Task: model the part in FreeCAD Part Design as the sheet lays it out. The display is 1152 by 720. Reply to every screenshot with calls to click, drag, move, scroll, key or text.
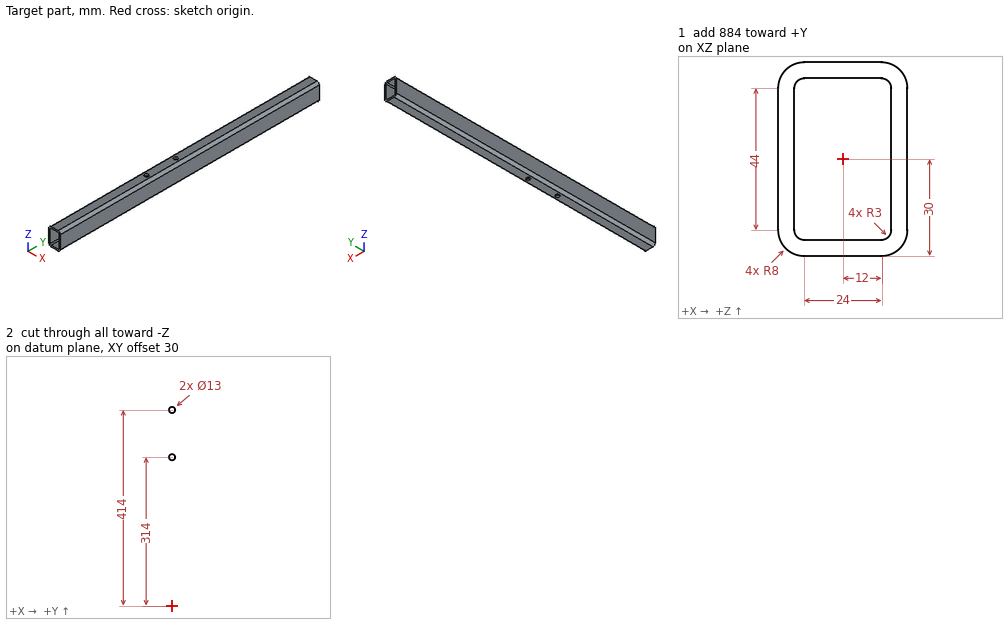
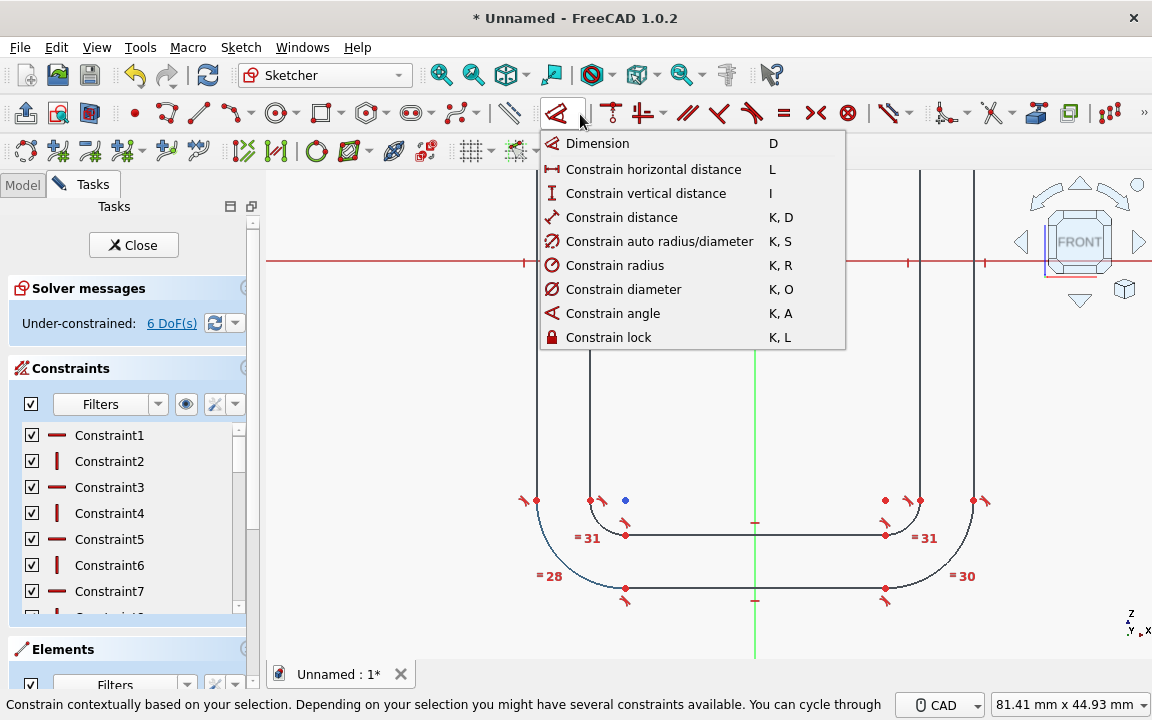
click(693, 265)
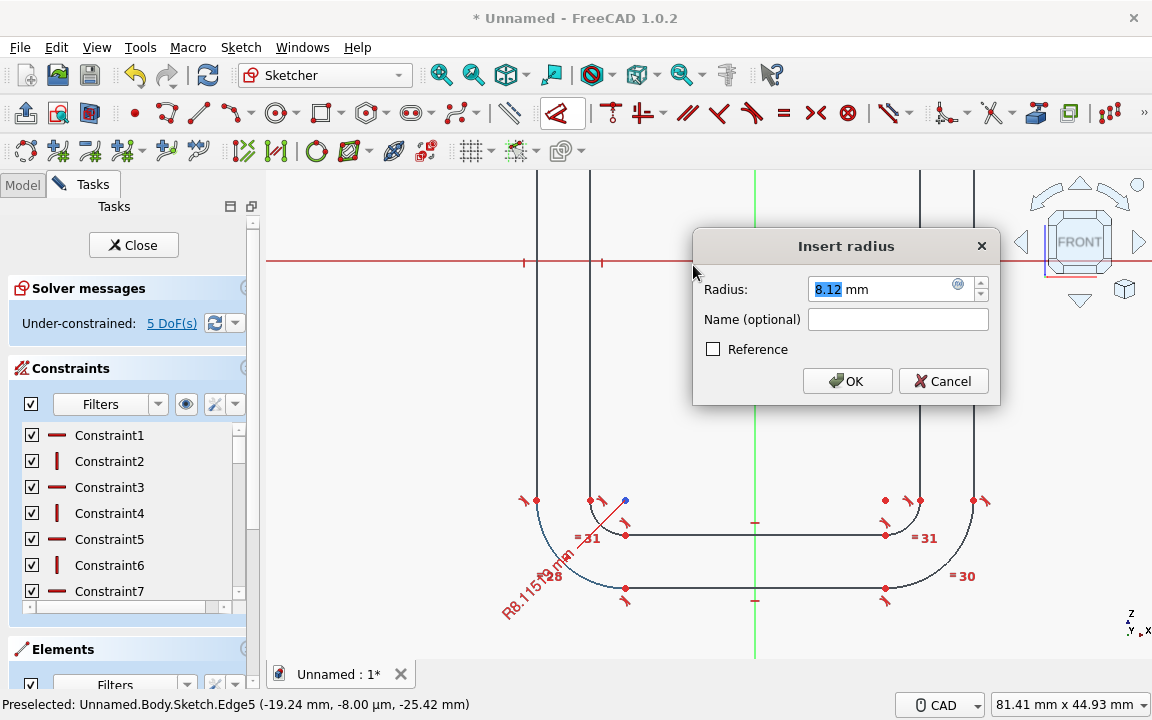
text(8)
key(Return)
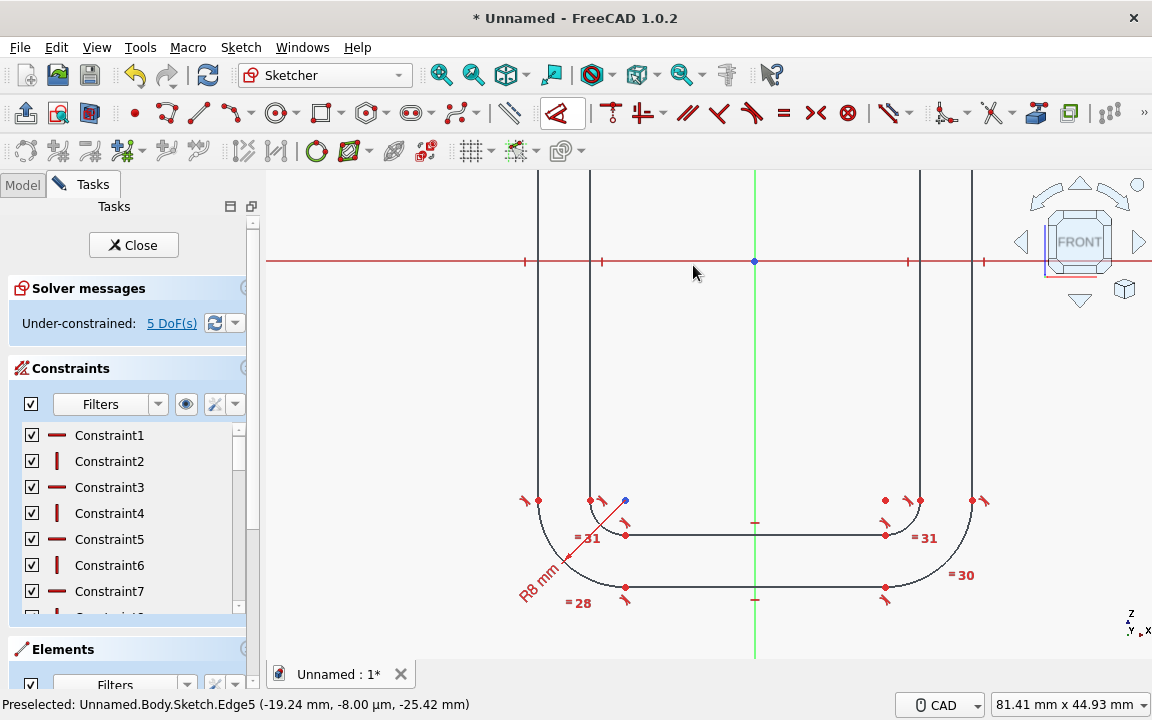
click(901, 531)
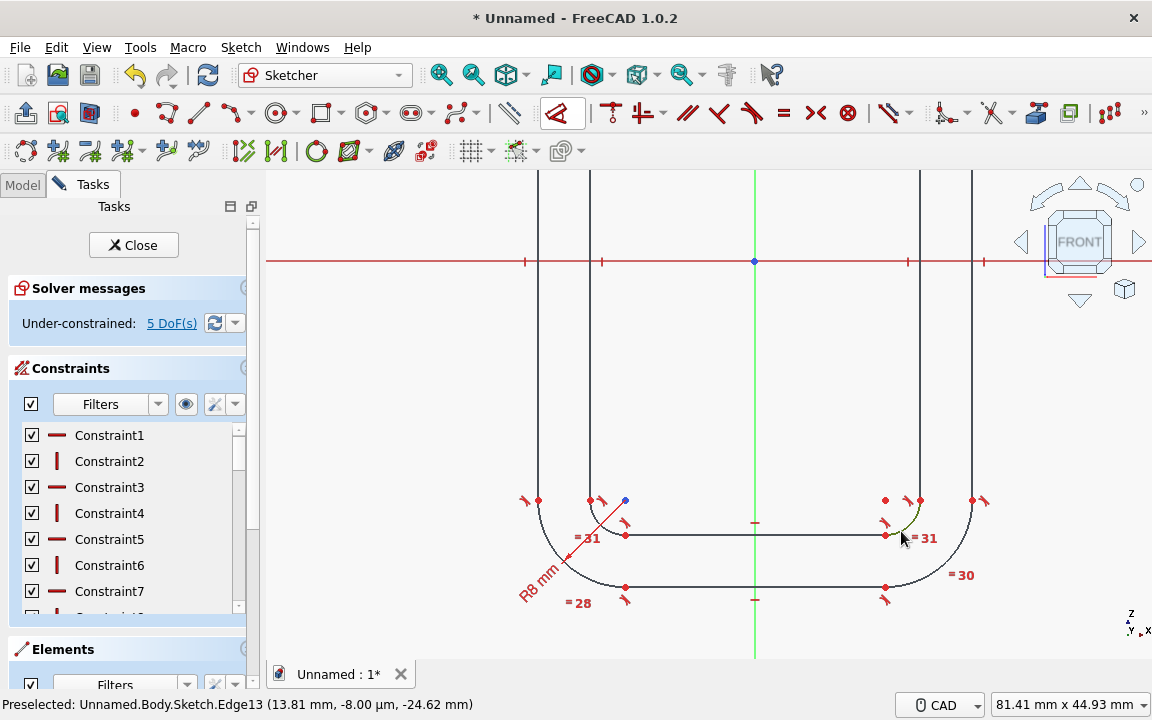
key(k)
key(r)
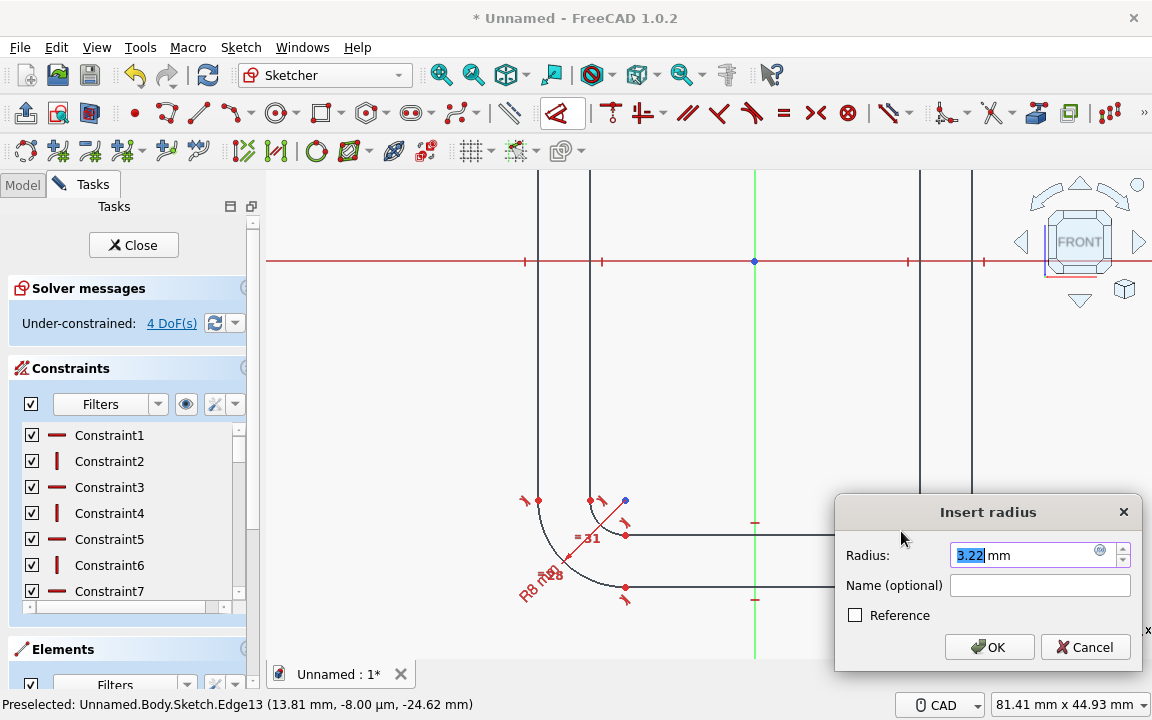
text(3)
key(Return)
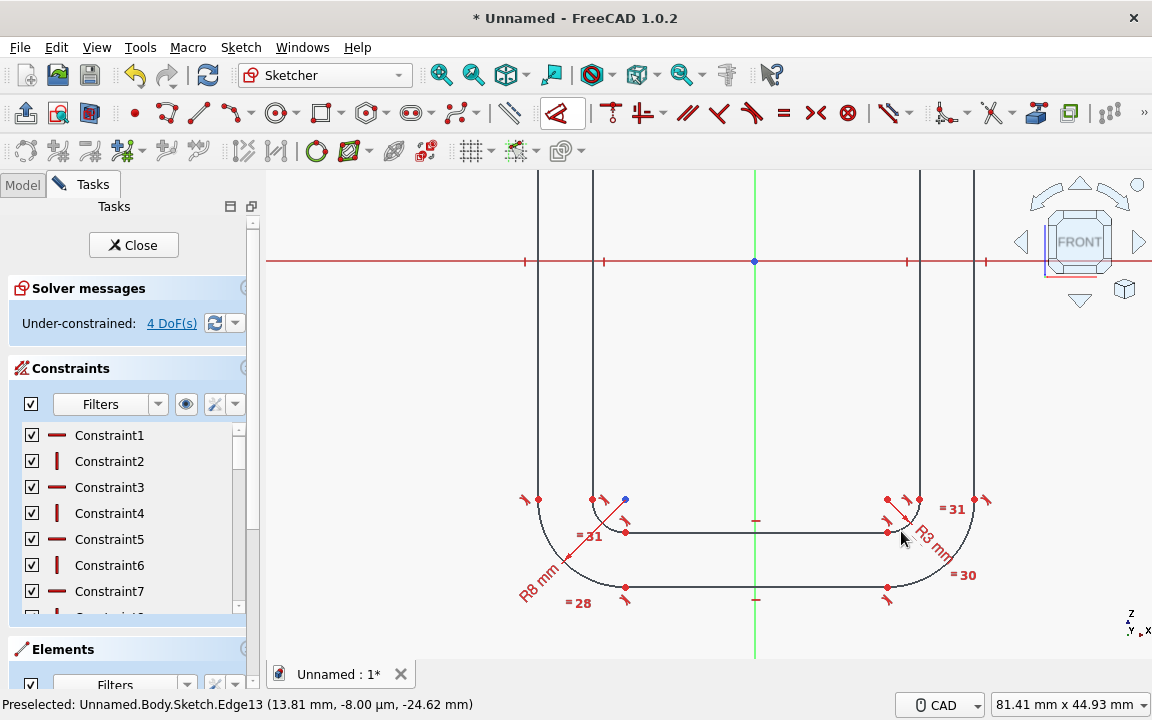
click(809, 587)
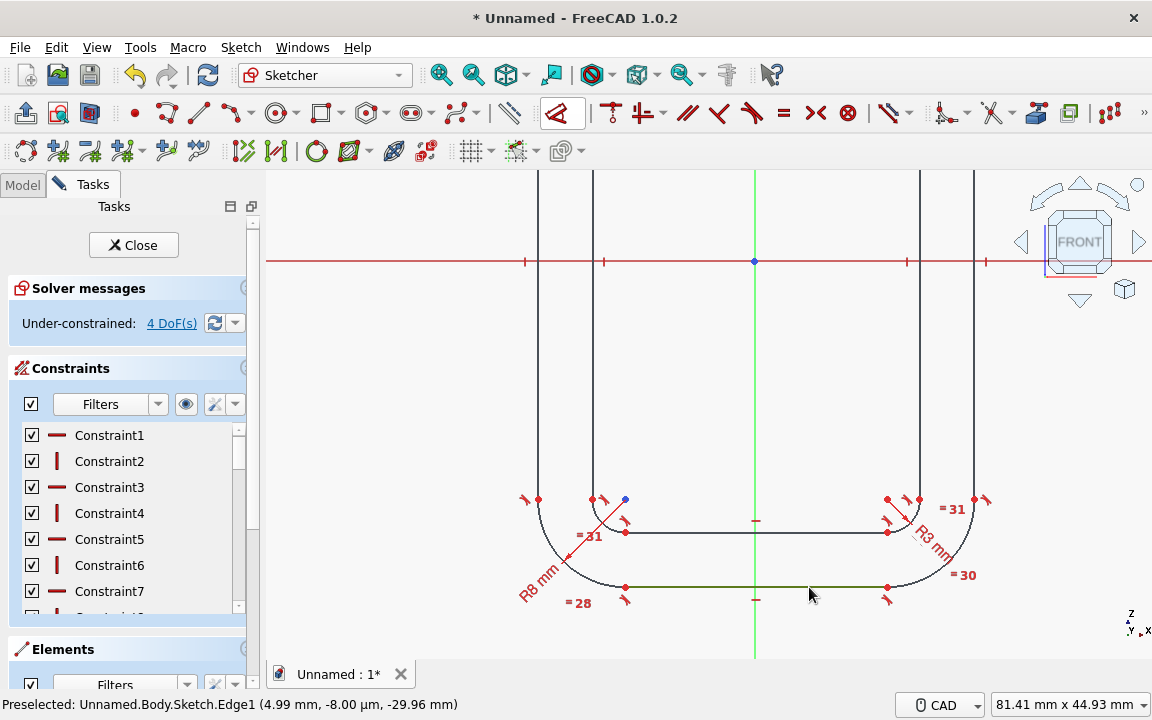
key(l)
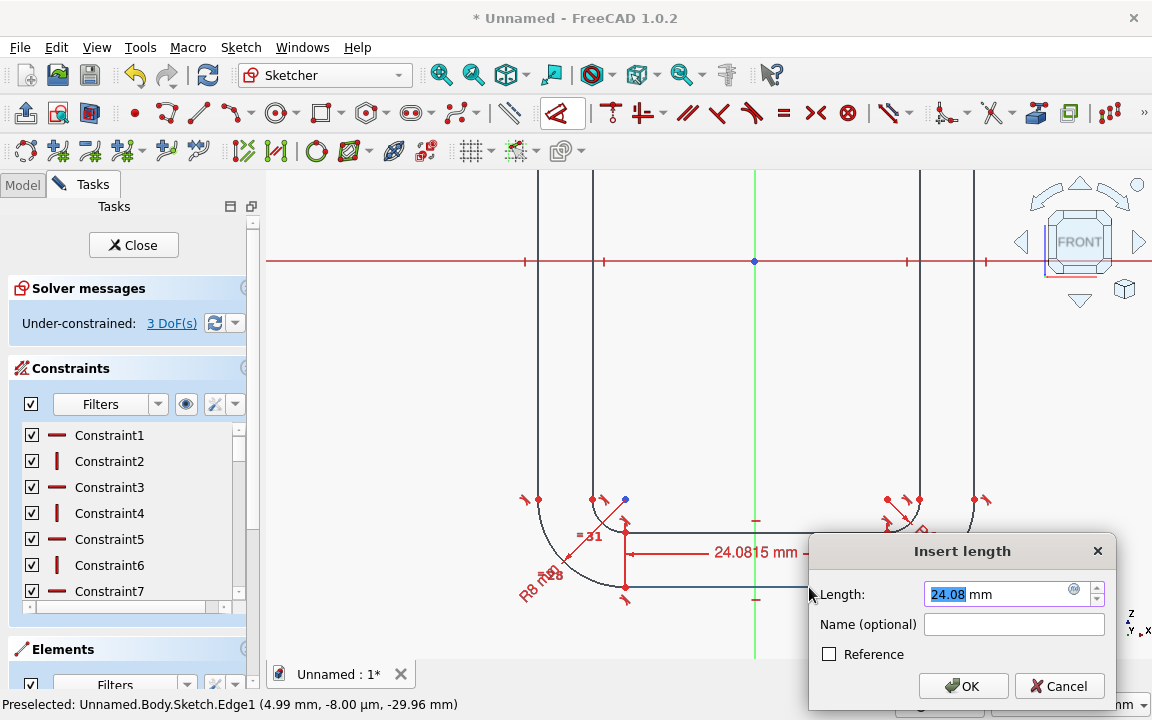
text(24)
key(Return)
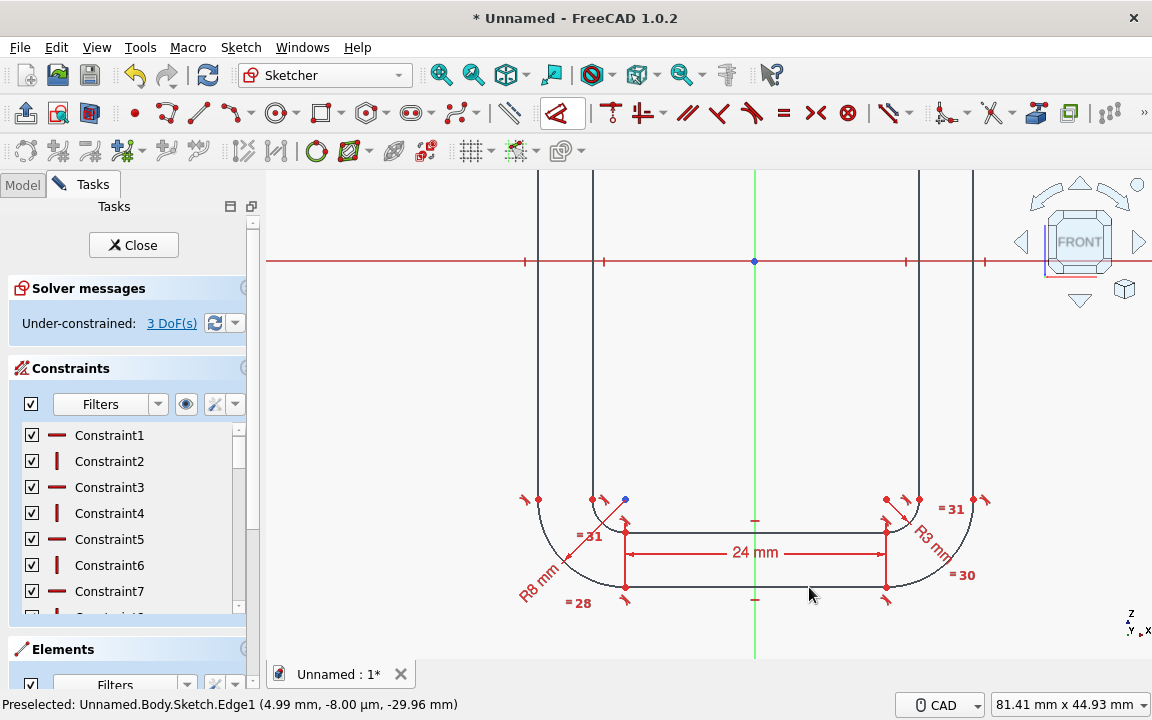
click(538, 357)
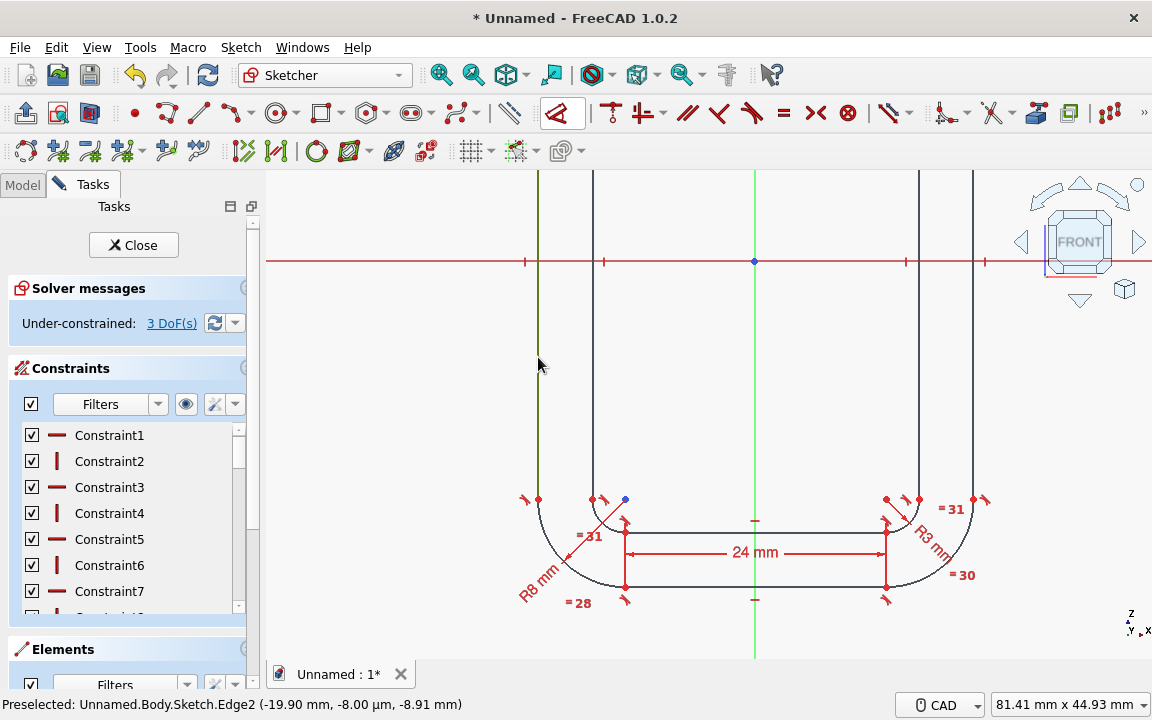
key(i)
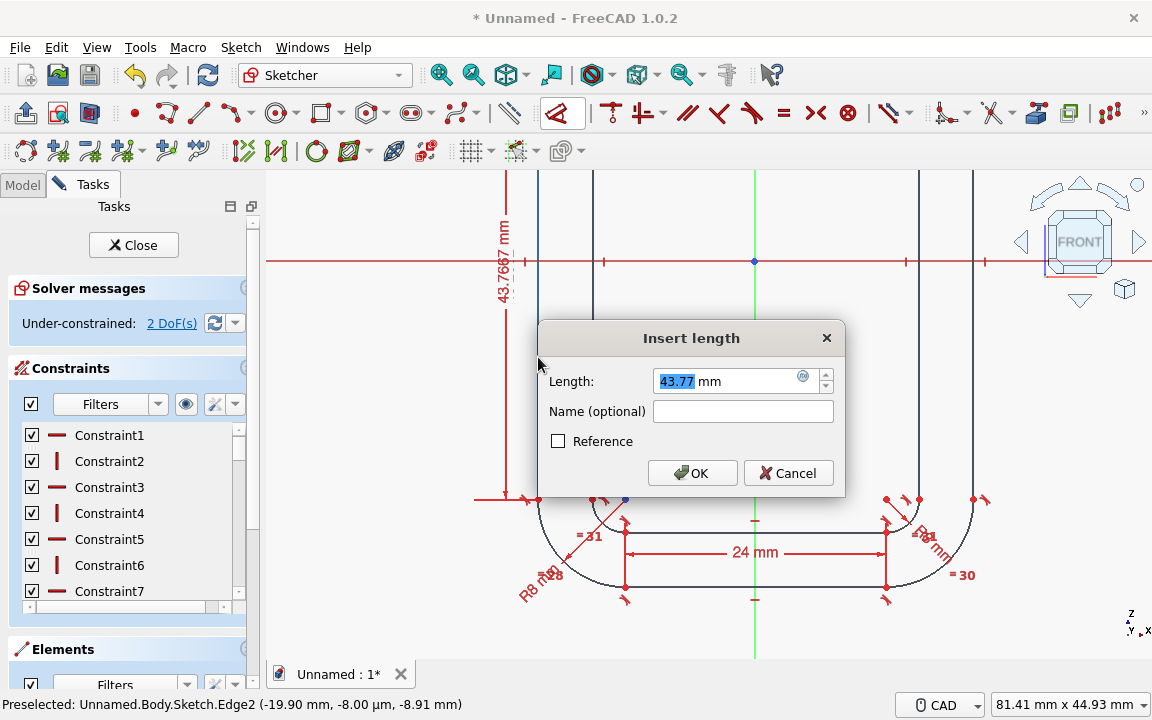
text(44)
key(Return)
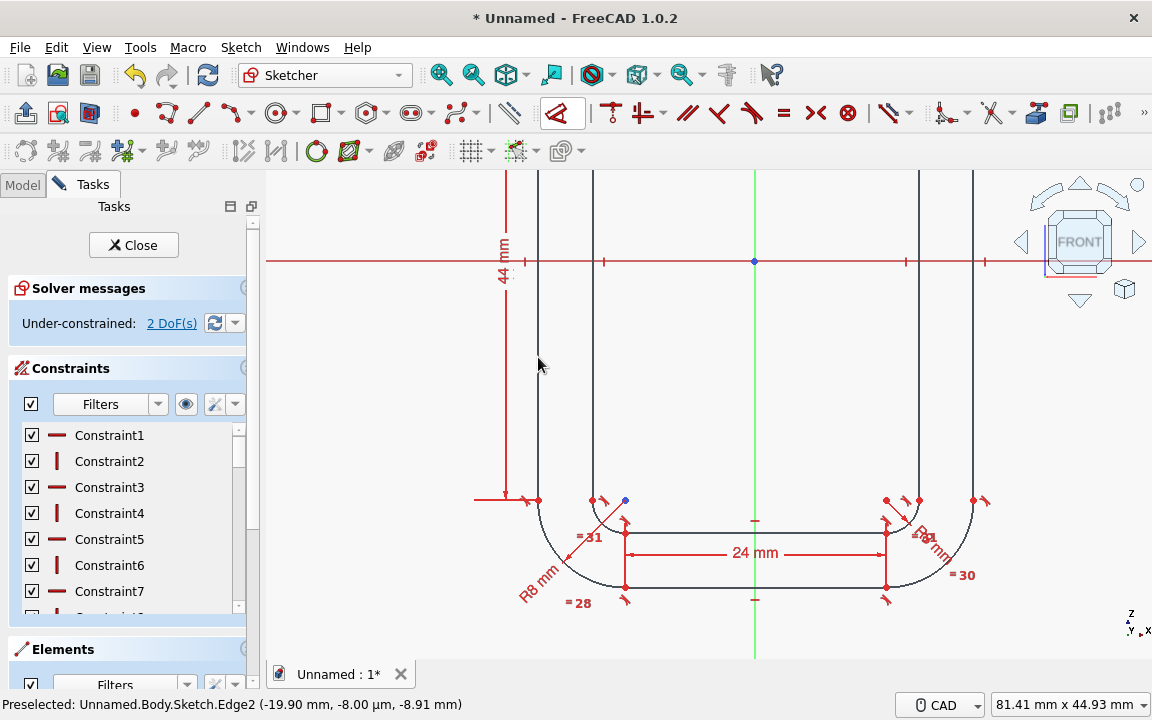
click(886, 588)